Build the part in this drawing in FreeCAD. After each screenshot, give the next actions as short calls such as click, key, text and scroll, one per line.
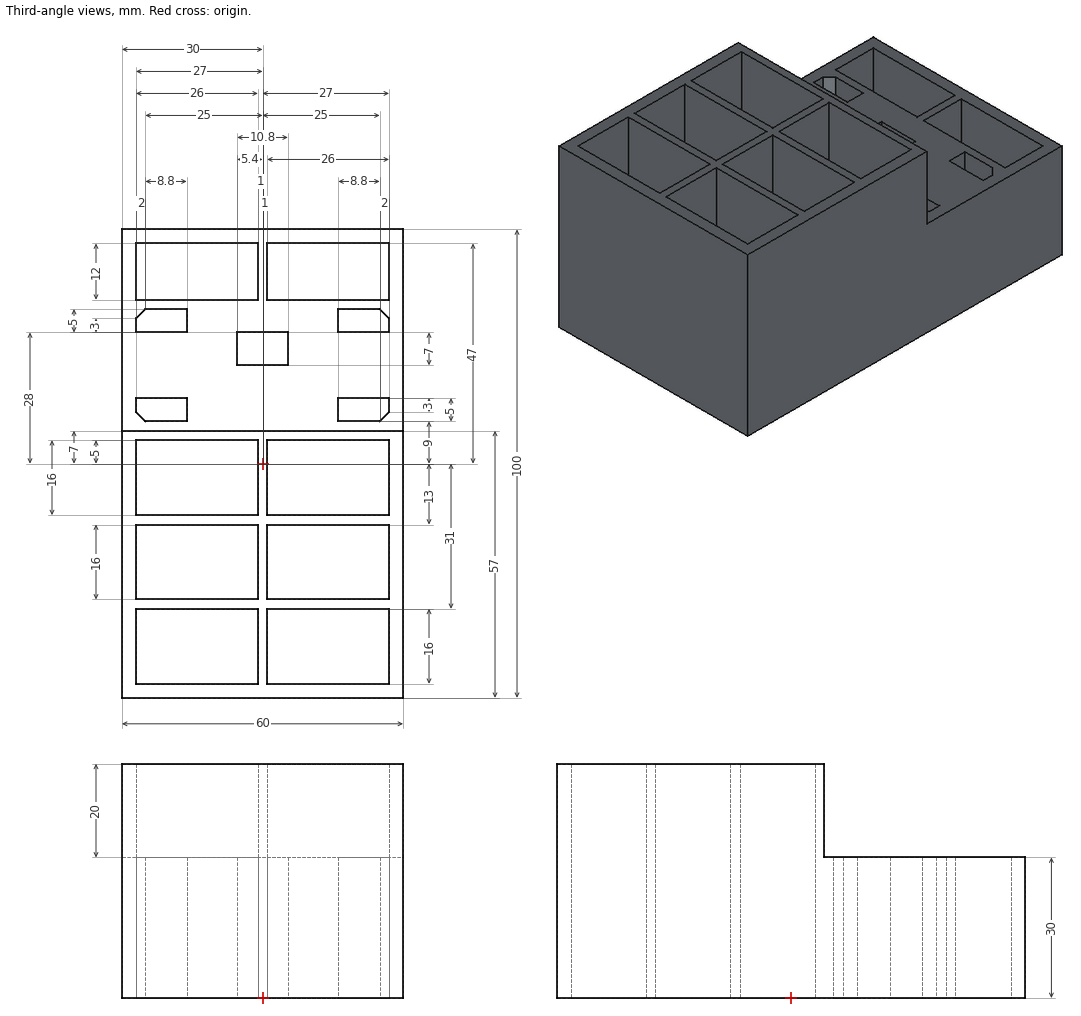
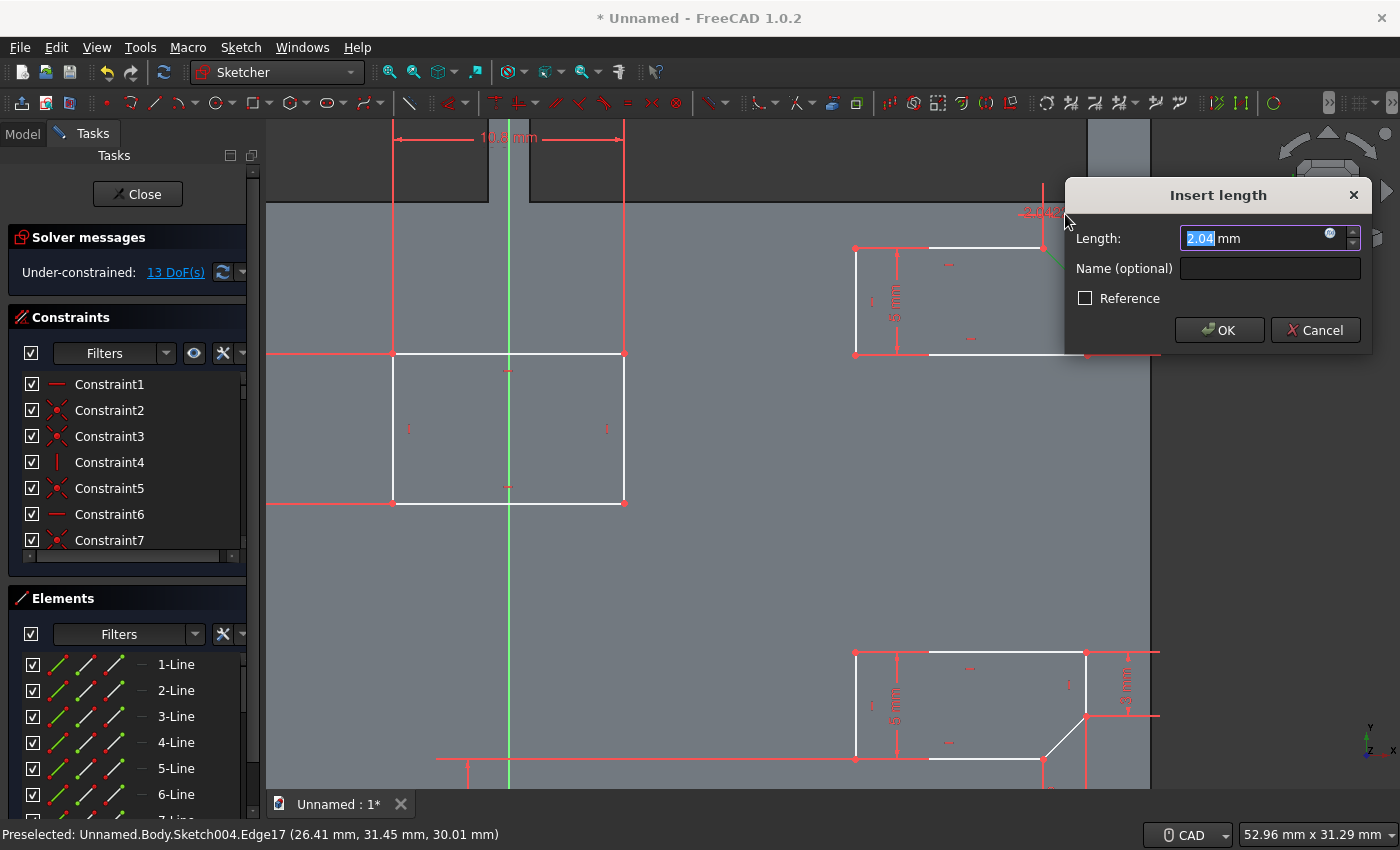
text(2)
key(Return)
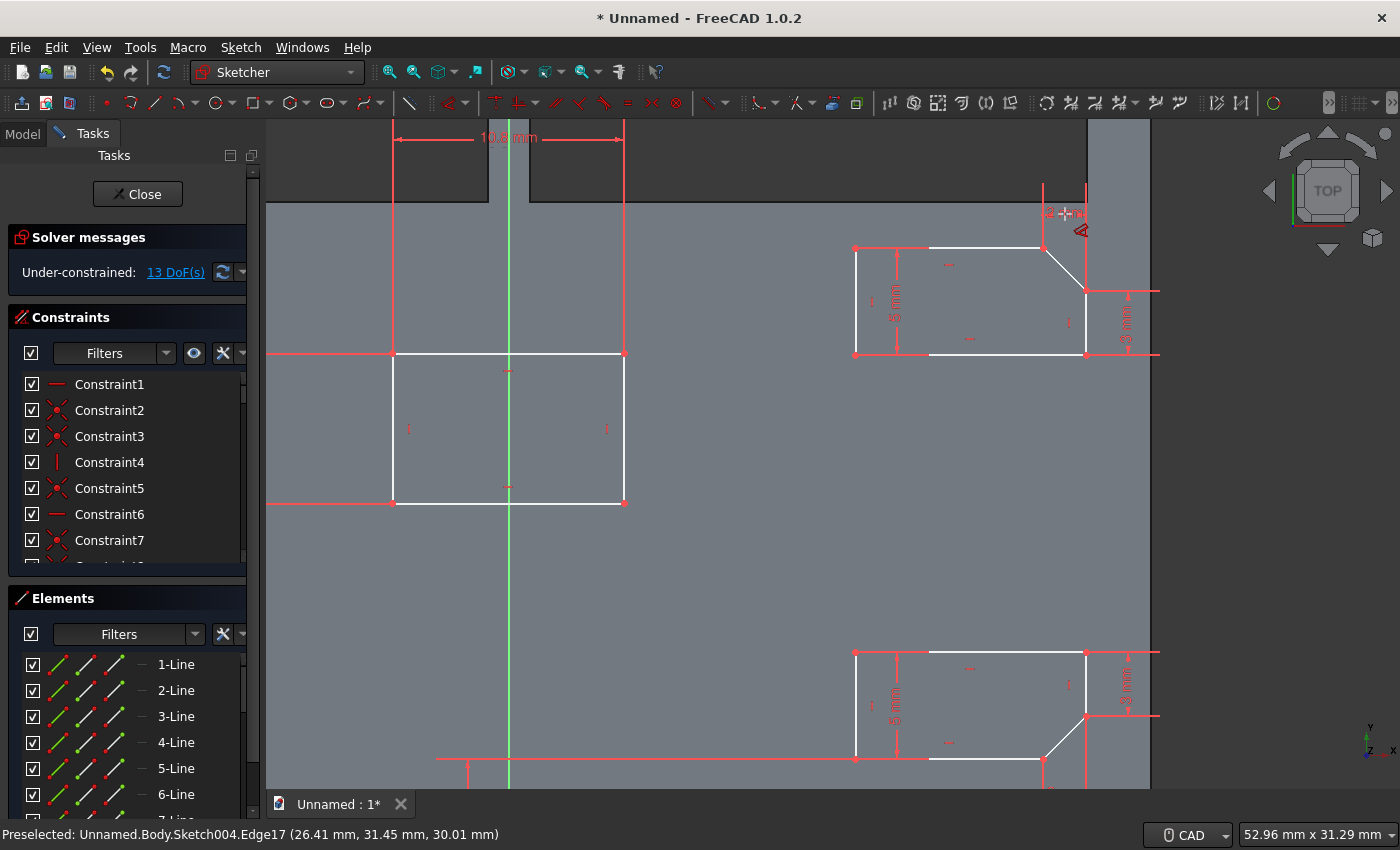
scroll(1075, 278, down, 3)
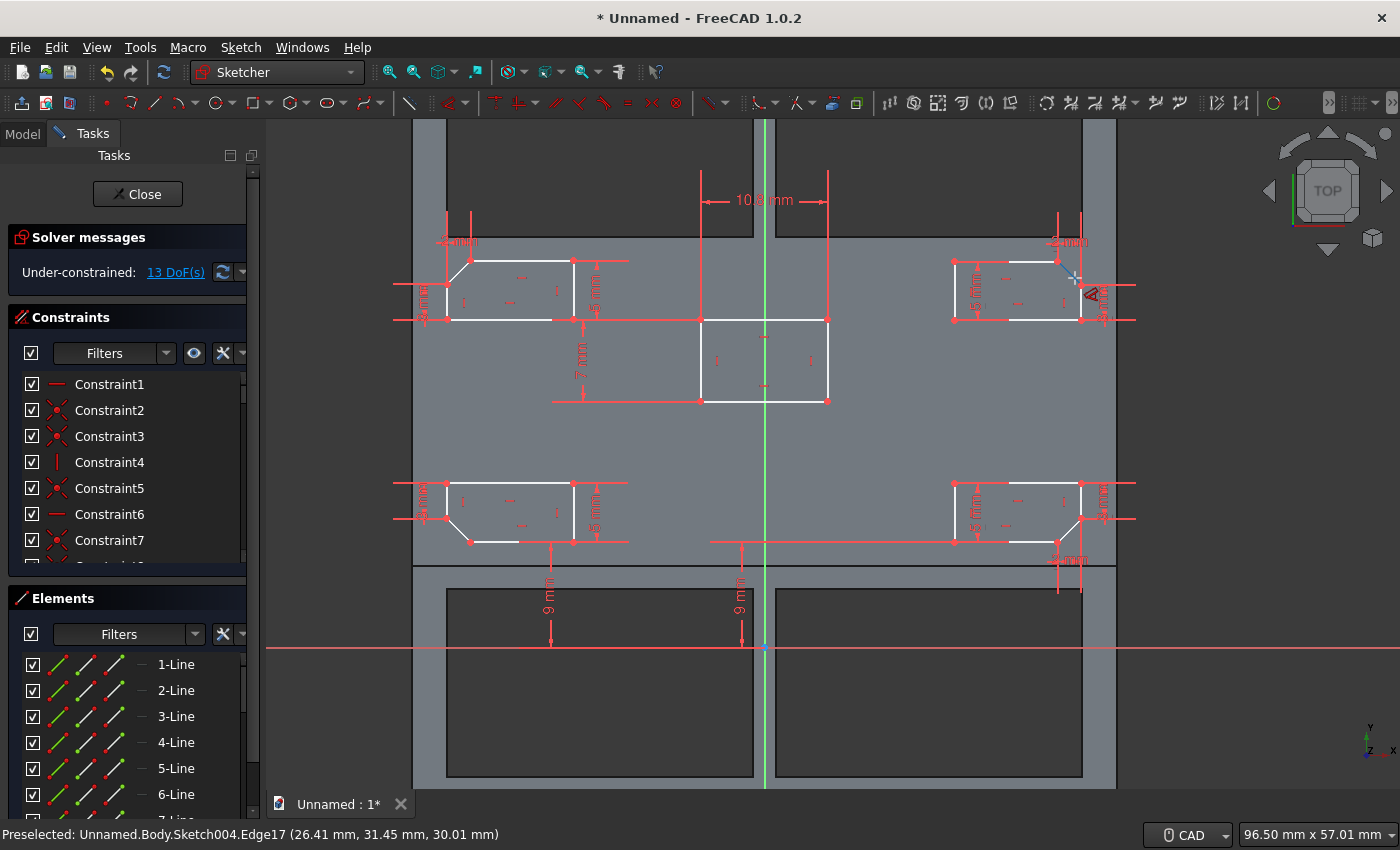
scroll(454, 526, up, 3)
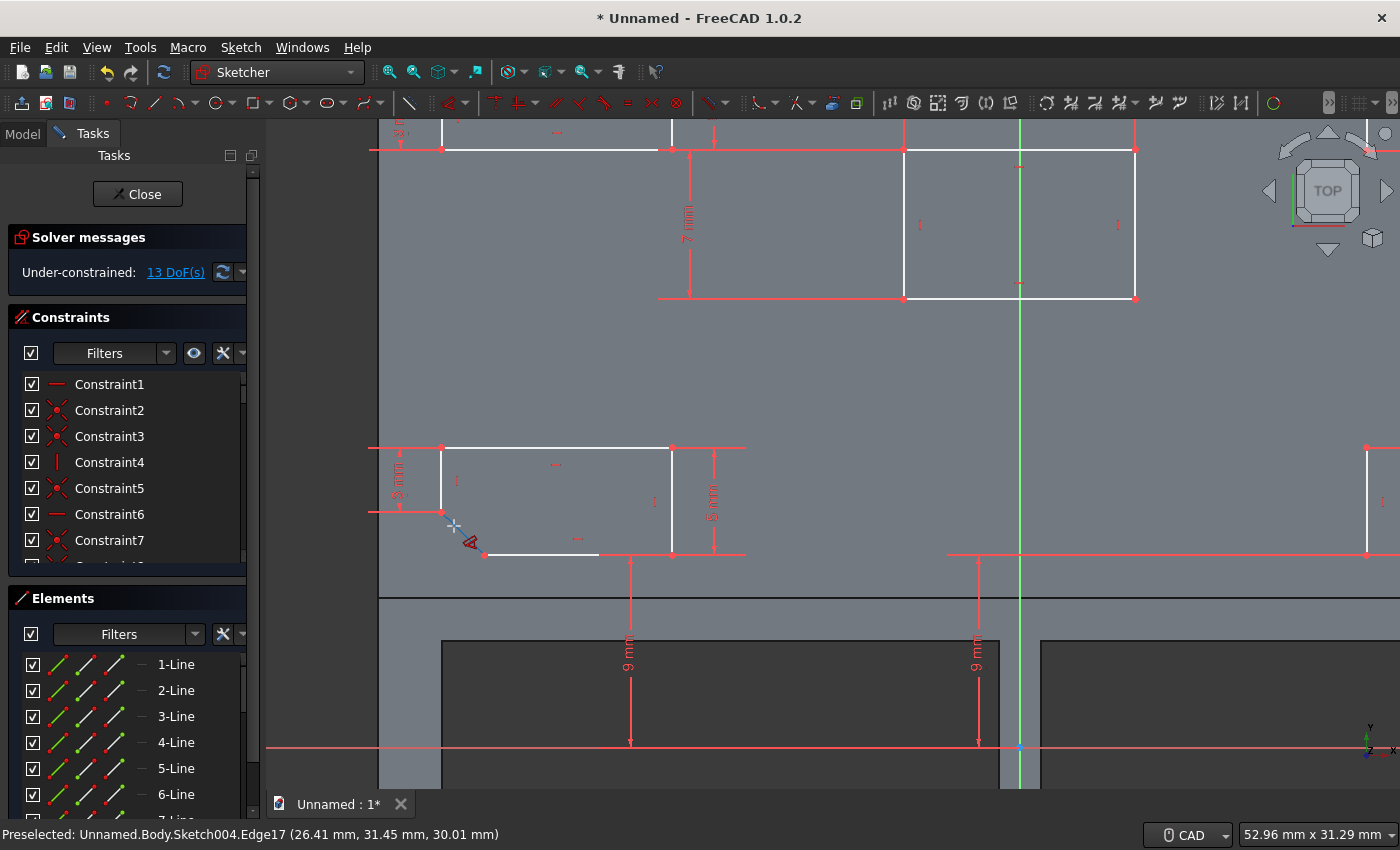
click(454, 525)
click(463, 589)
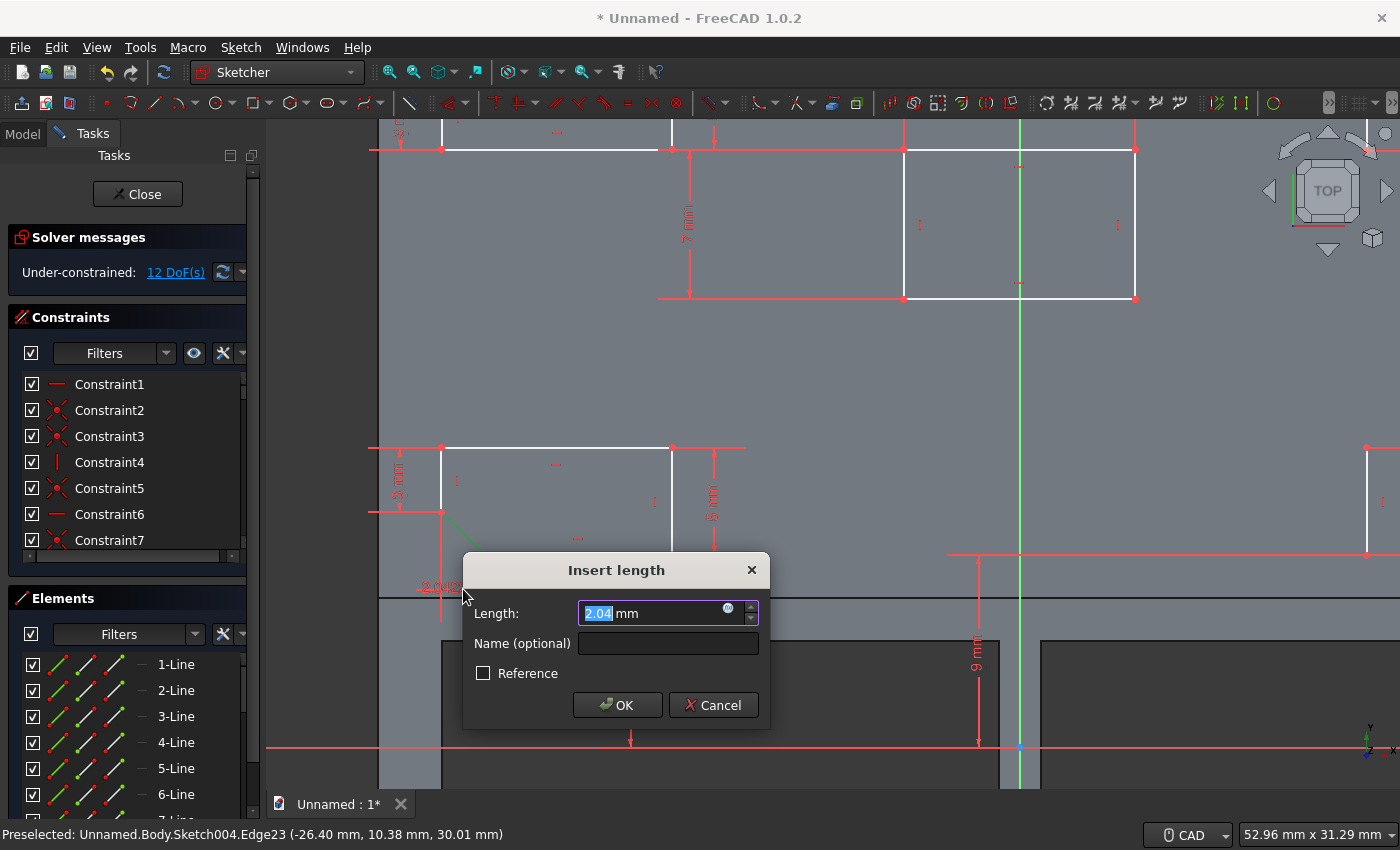
text(2)
key(Return)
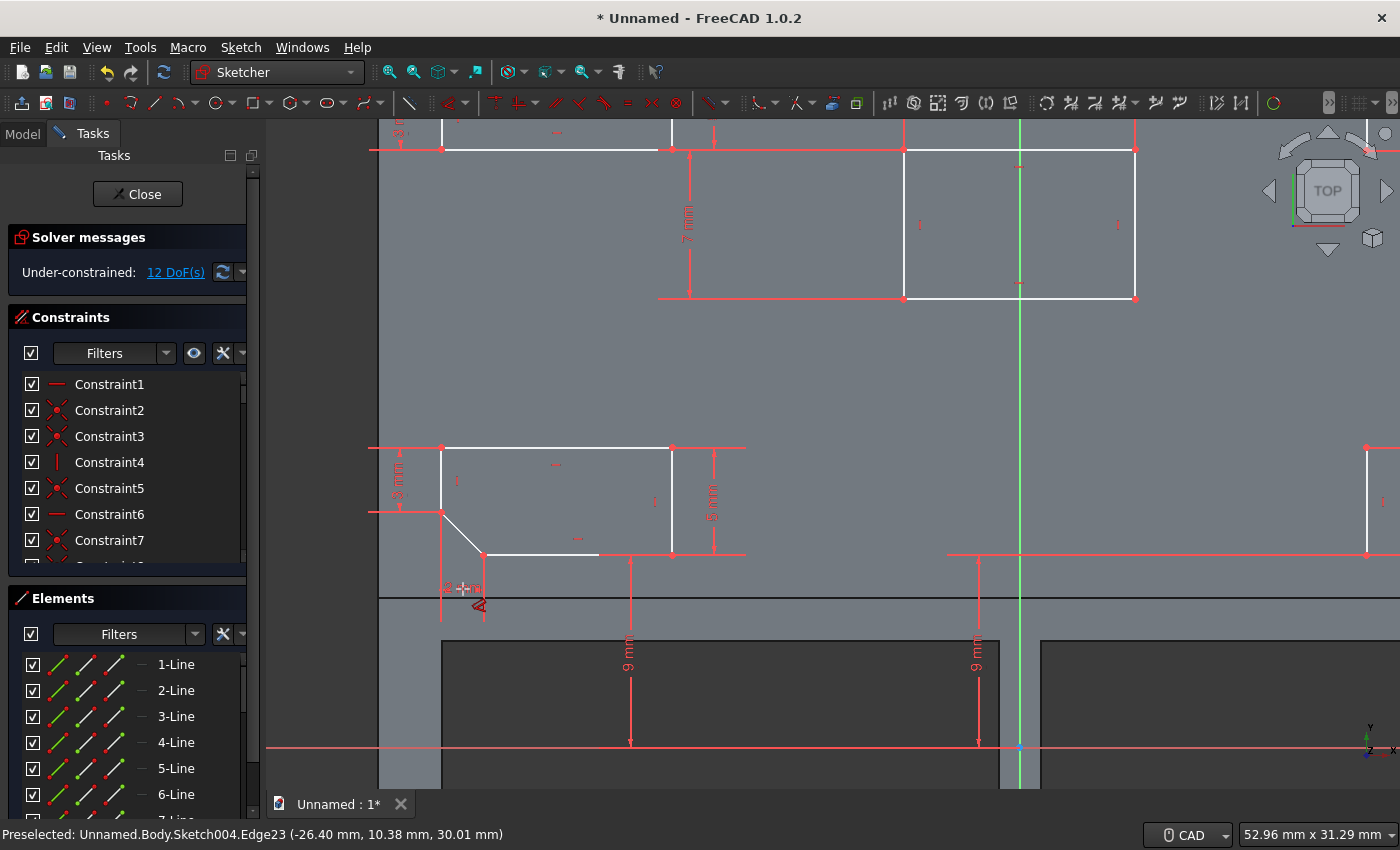
scroll(454, 526, down, 3)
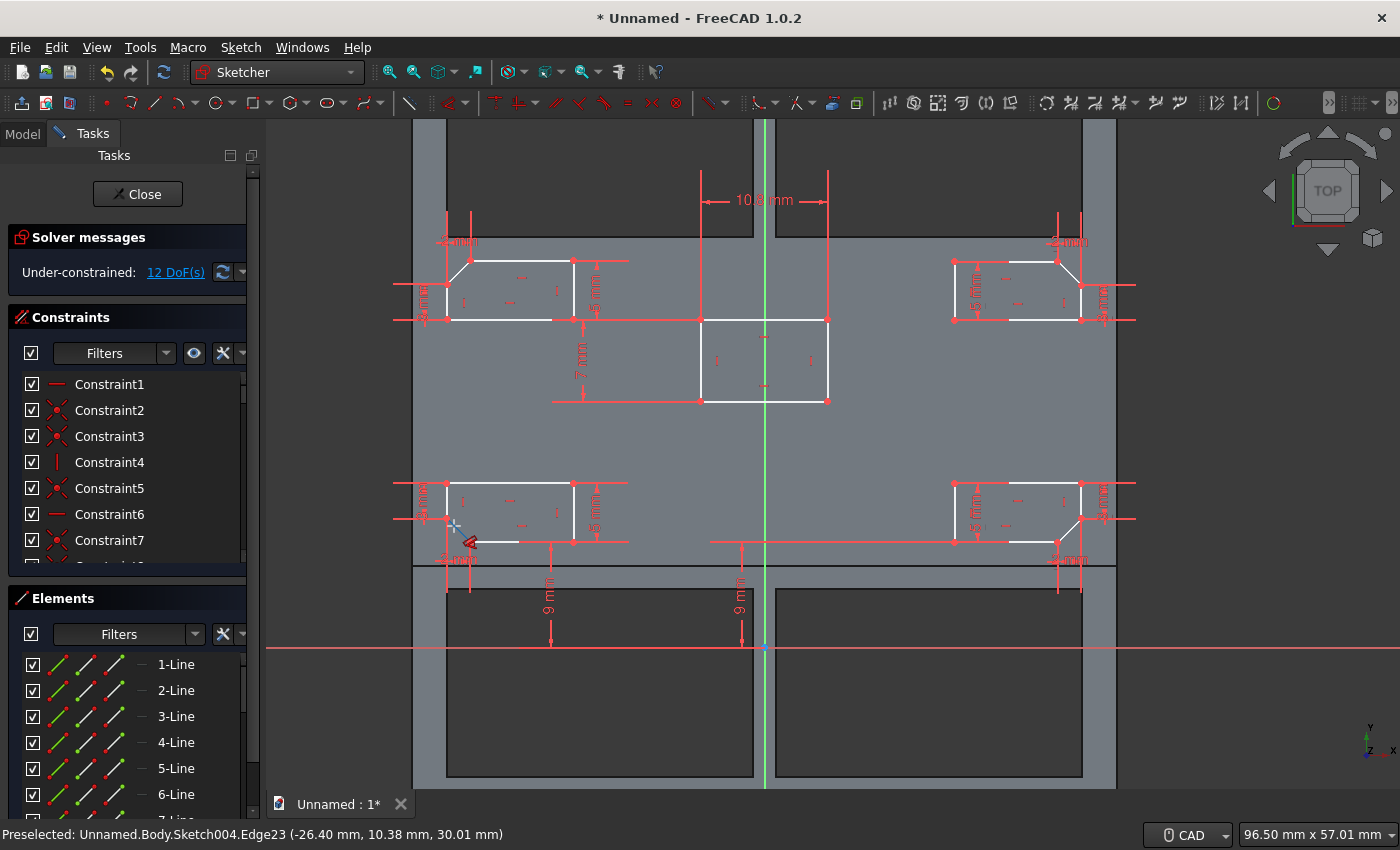
click(986, 542)
click(983, 576)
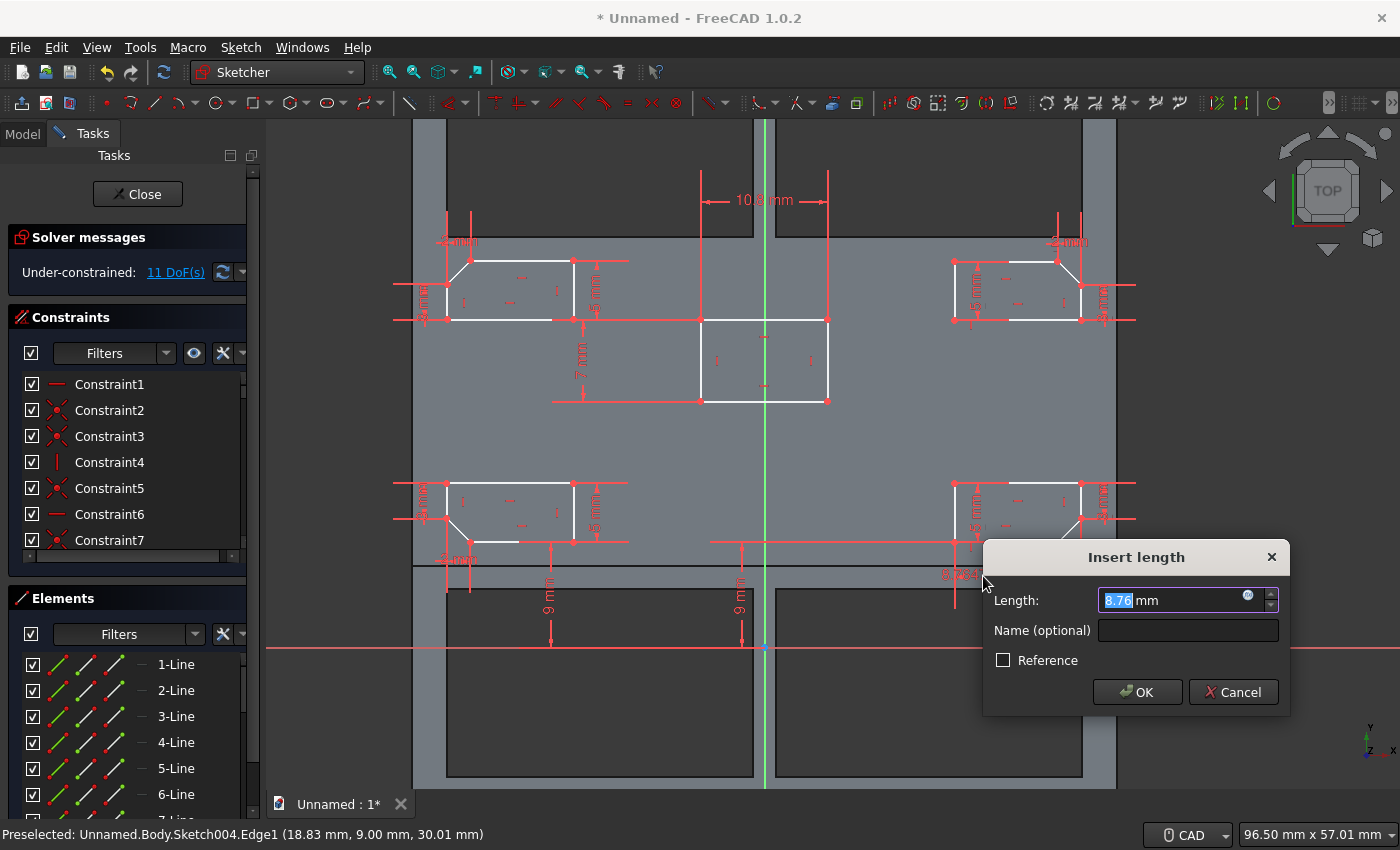
text(8.8)
key(Return)